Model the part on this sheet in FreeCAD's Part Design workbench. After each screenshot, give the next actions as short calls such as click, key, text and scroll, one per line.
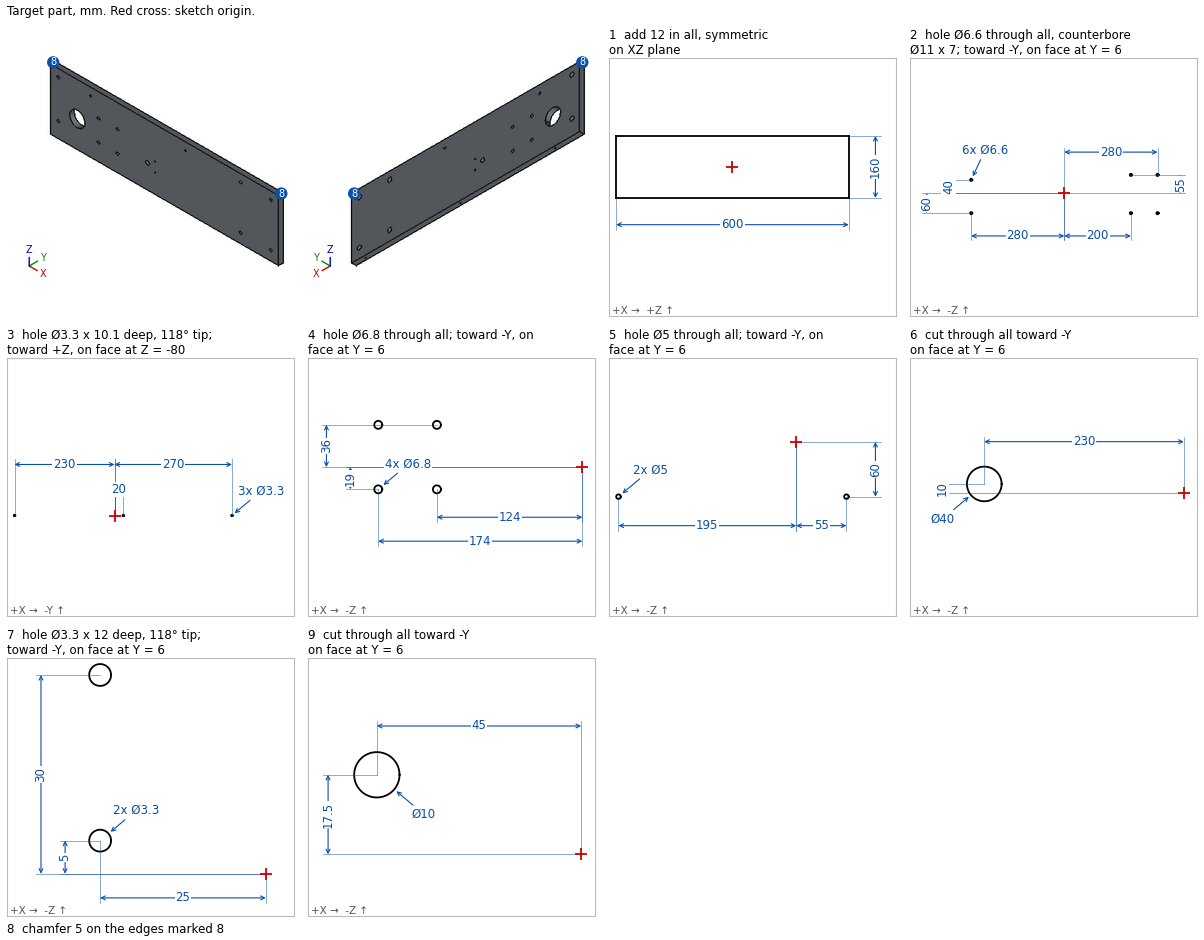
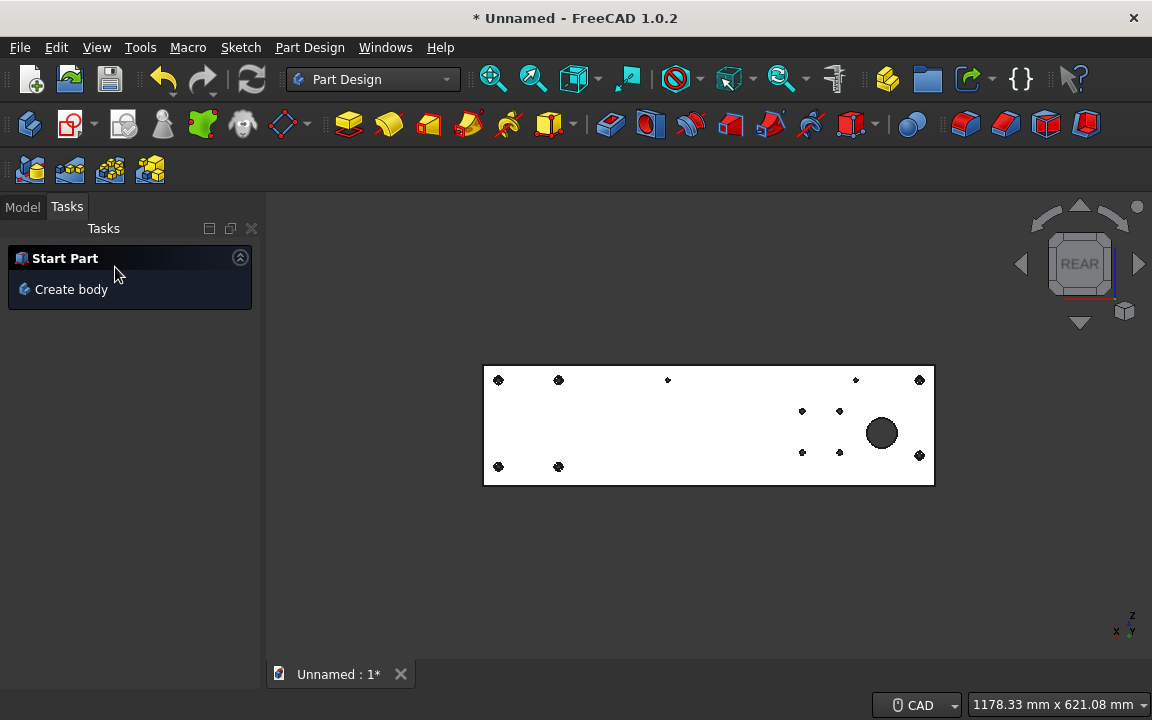
click(709, 424)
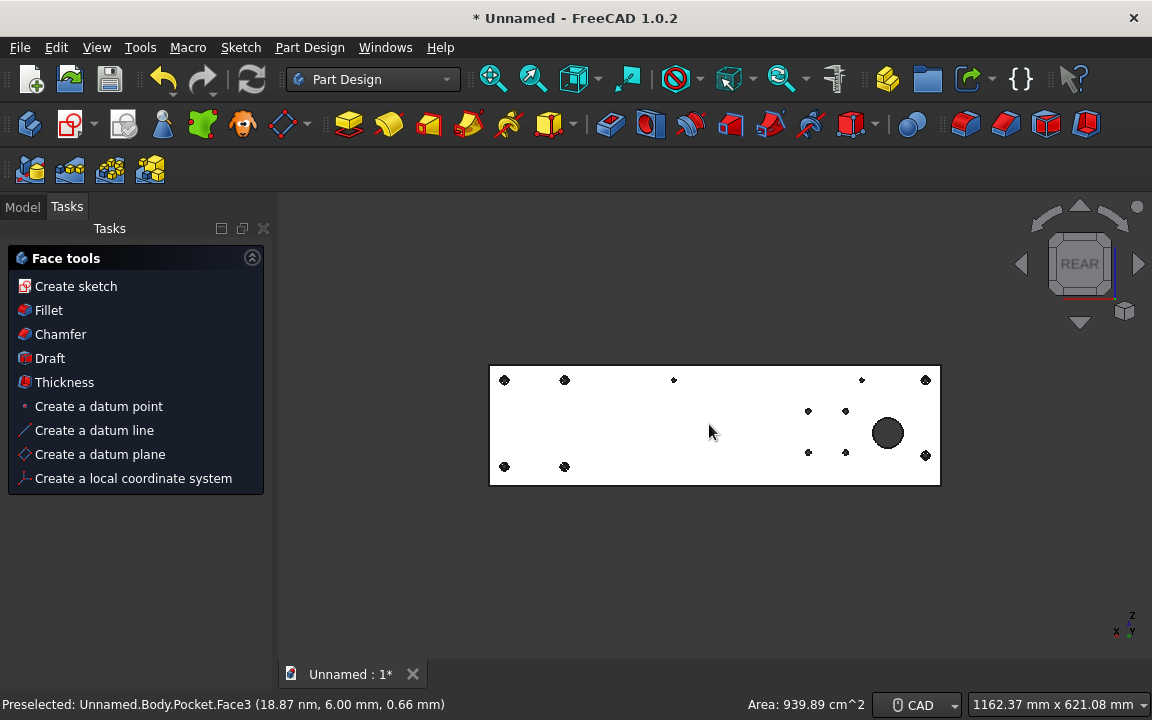
click(70, 124)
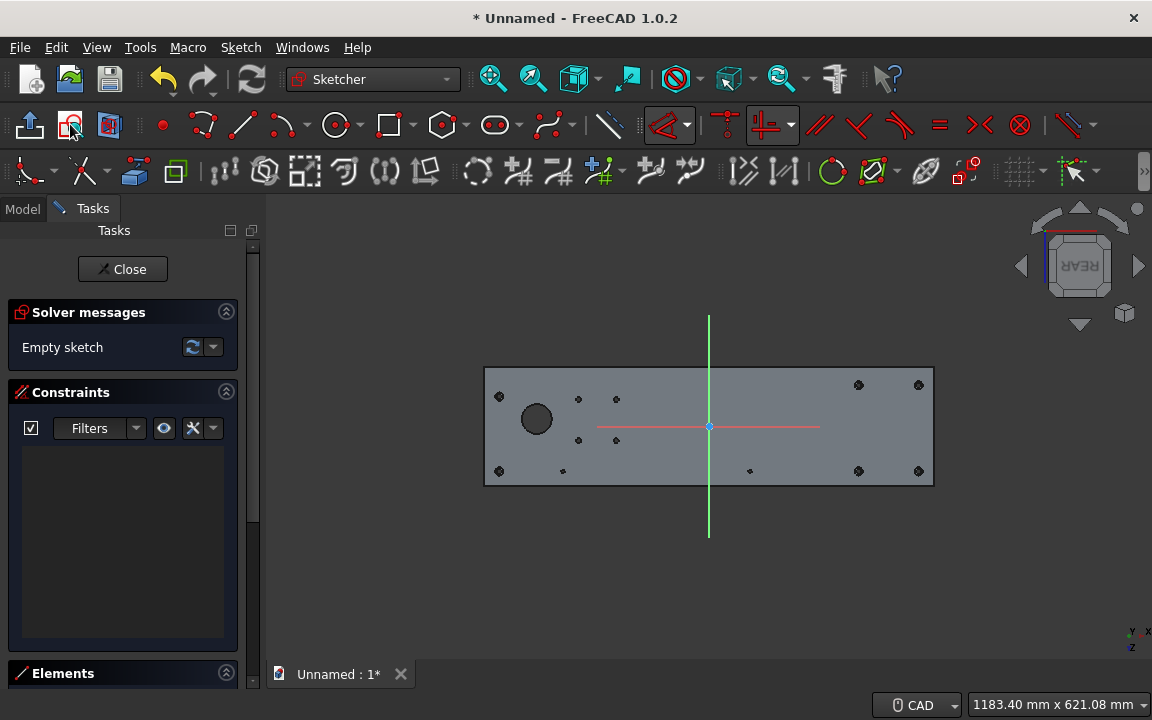
scroll(705, 413, up, 12)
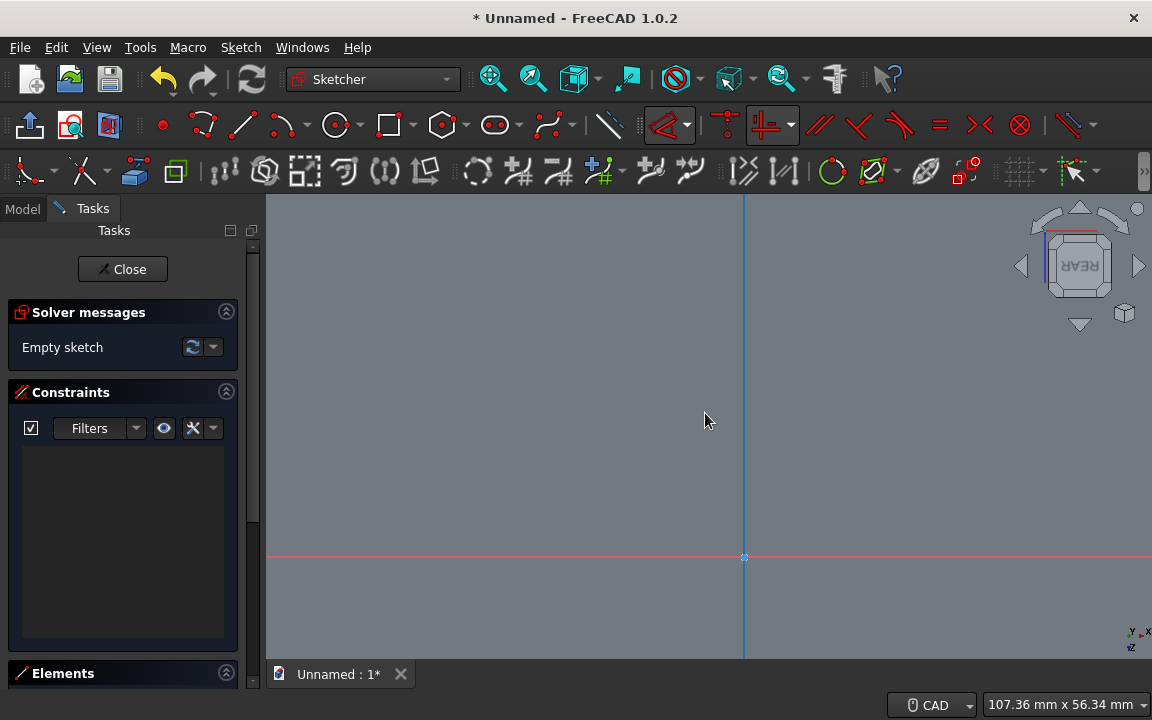
click(336, 126)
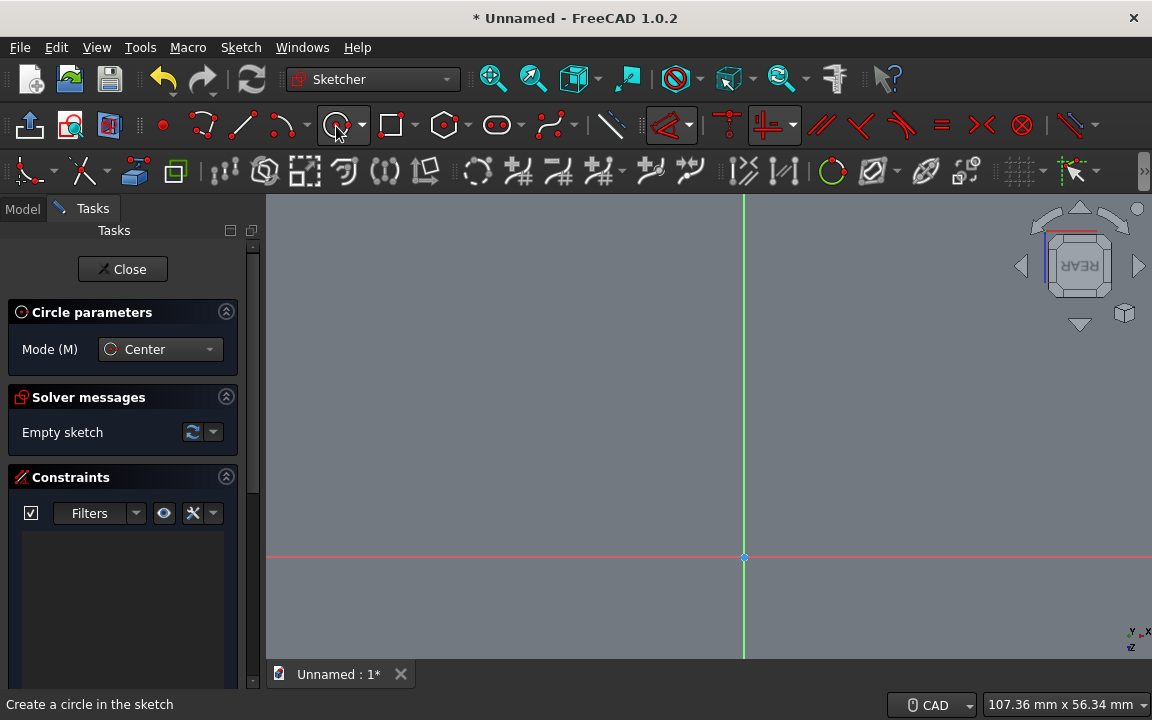
scroll(538, 516, up, 3)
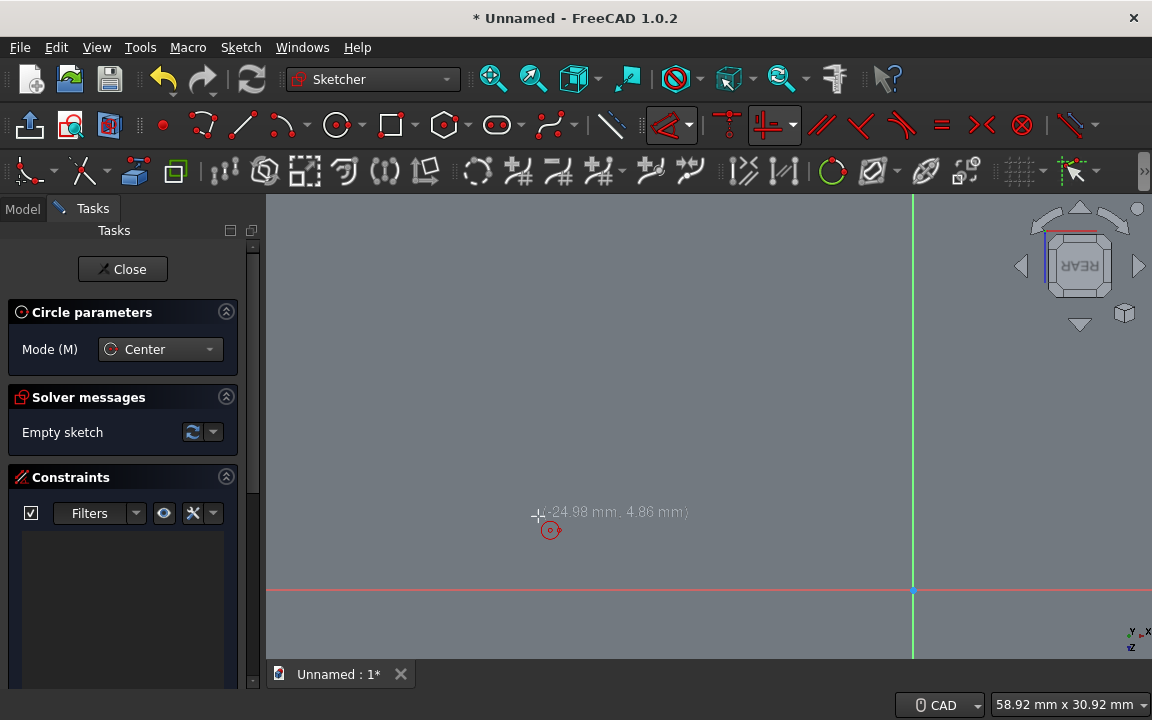
click(537, 515)
move(555, 498)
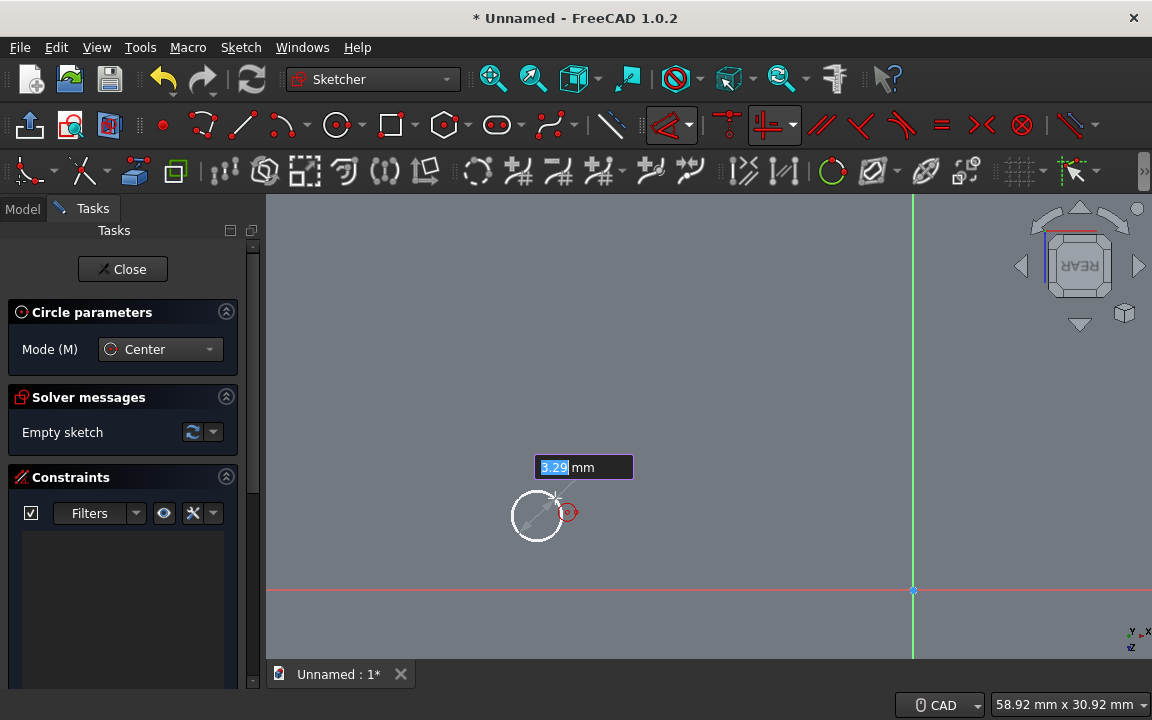
text(3.3)
key(Return)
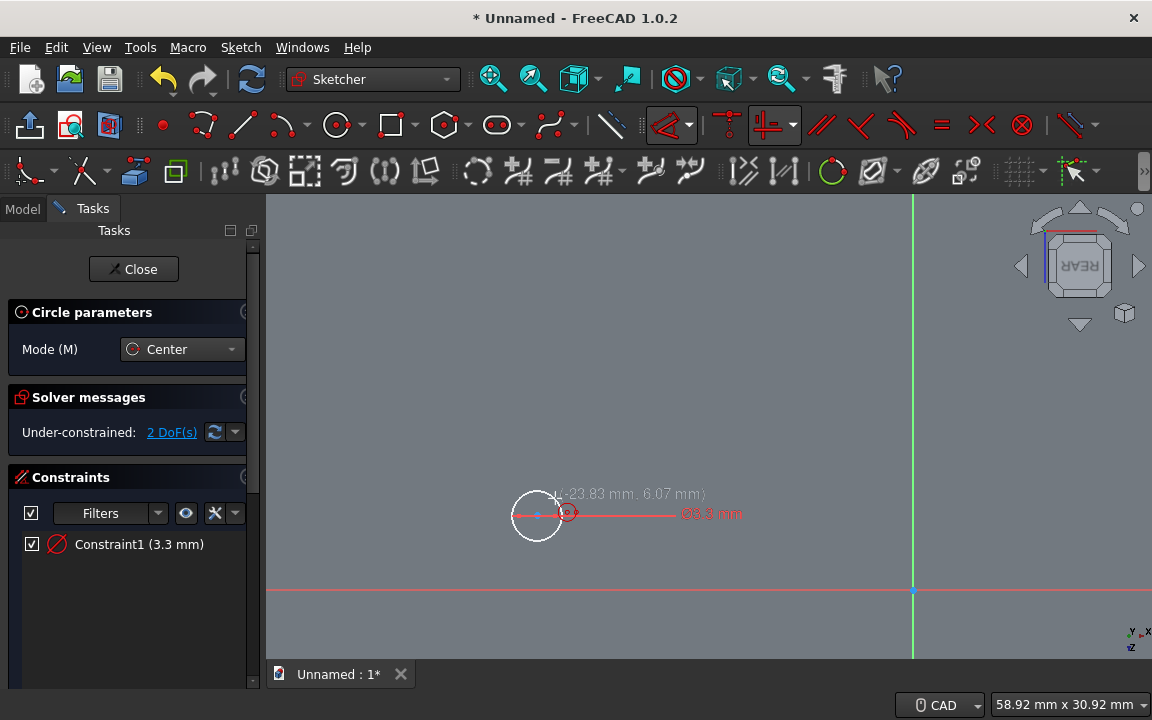
scroll(552, 517, down, 3)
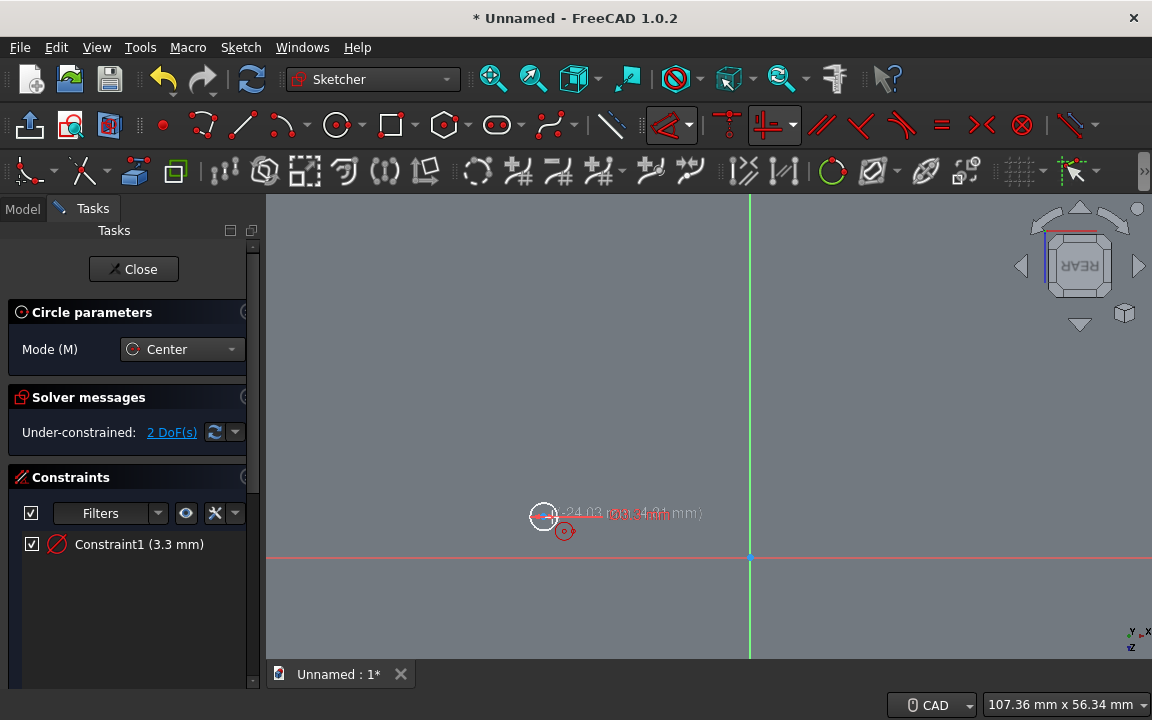
scroll(544, 310, up, 3)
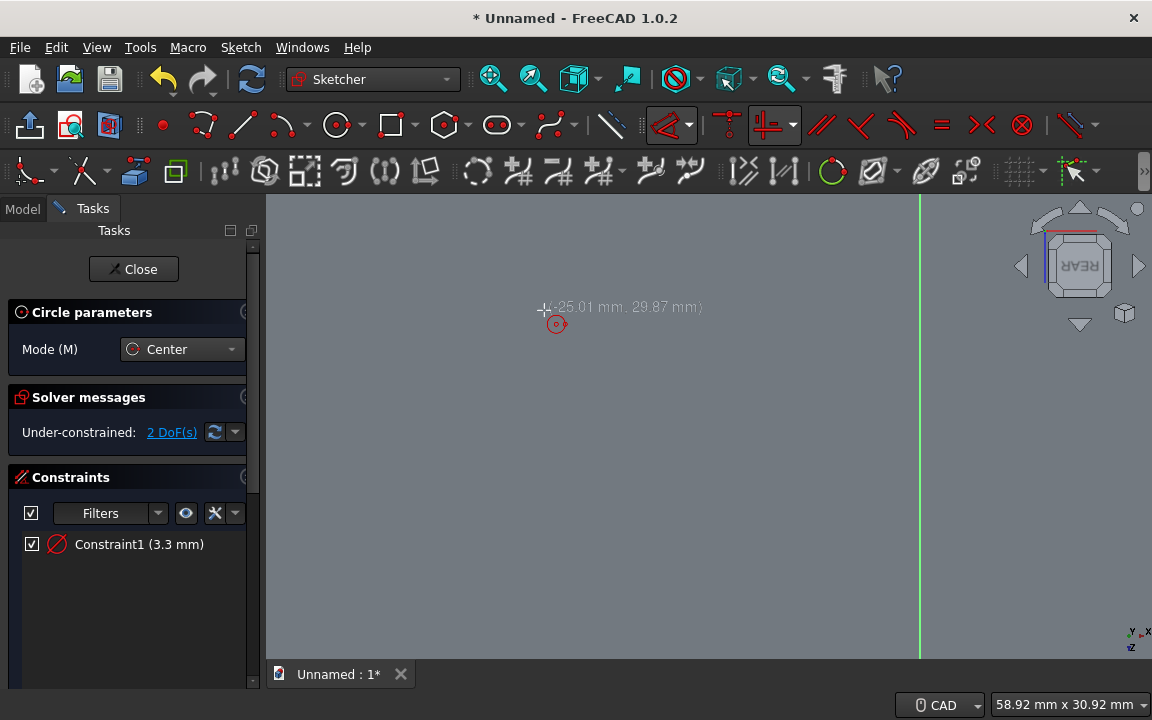
click(544, 310)
move(562, 292)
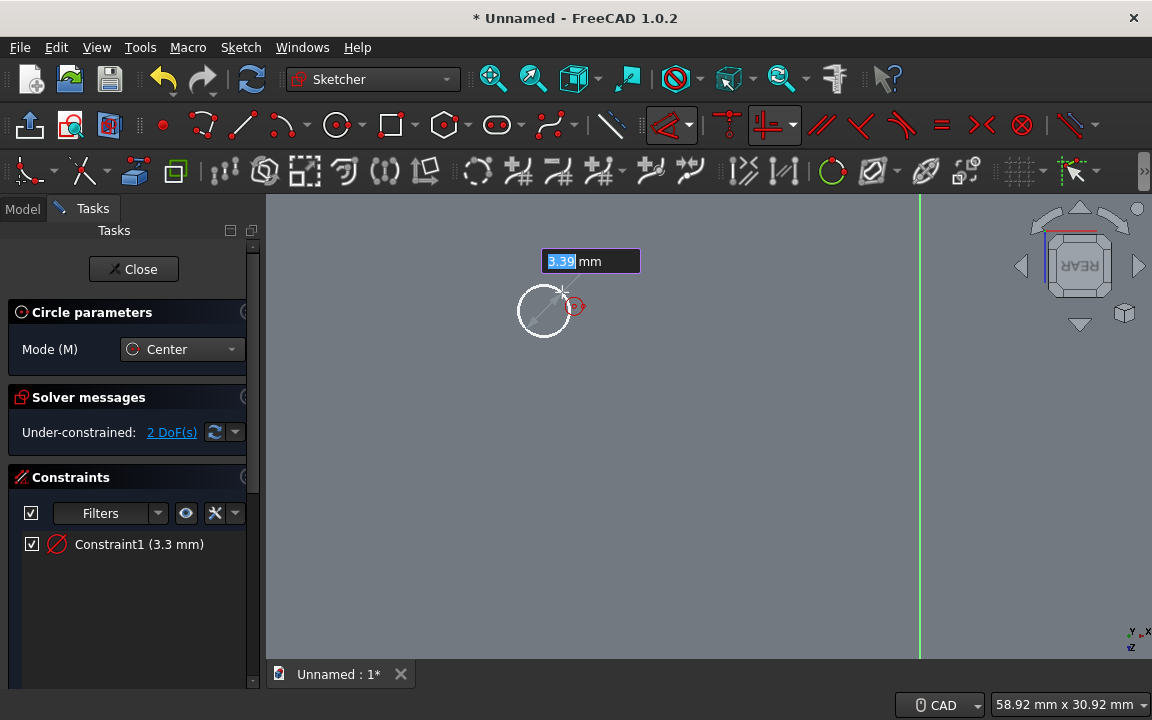
text(3.3)
key(Return)
key(Escape)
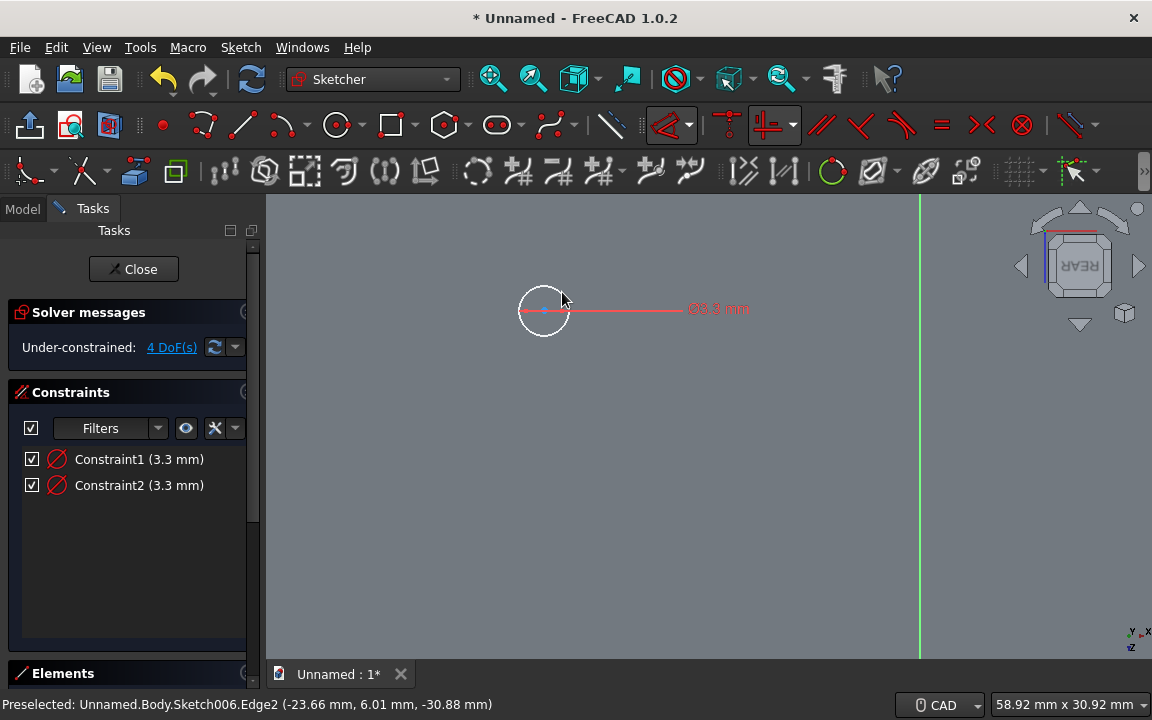
scroll(544, 309, down, 3)